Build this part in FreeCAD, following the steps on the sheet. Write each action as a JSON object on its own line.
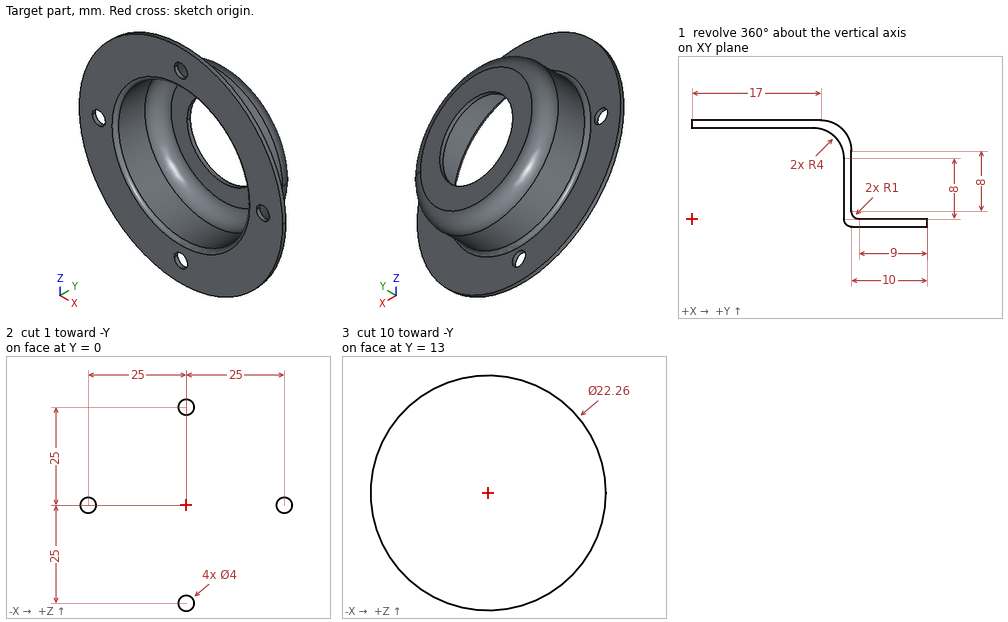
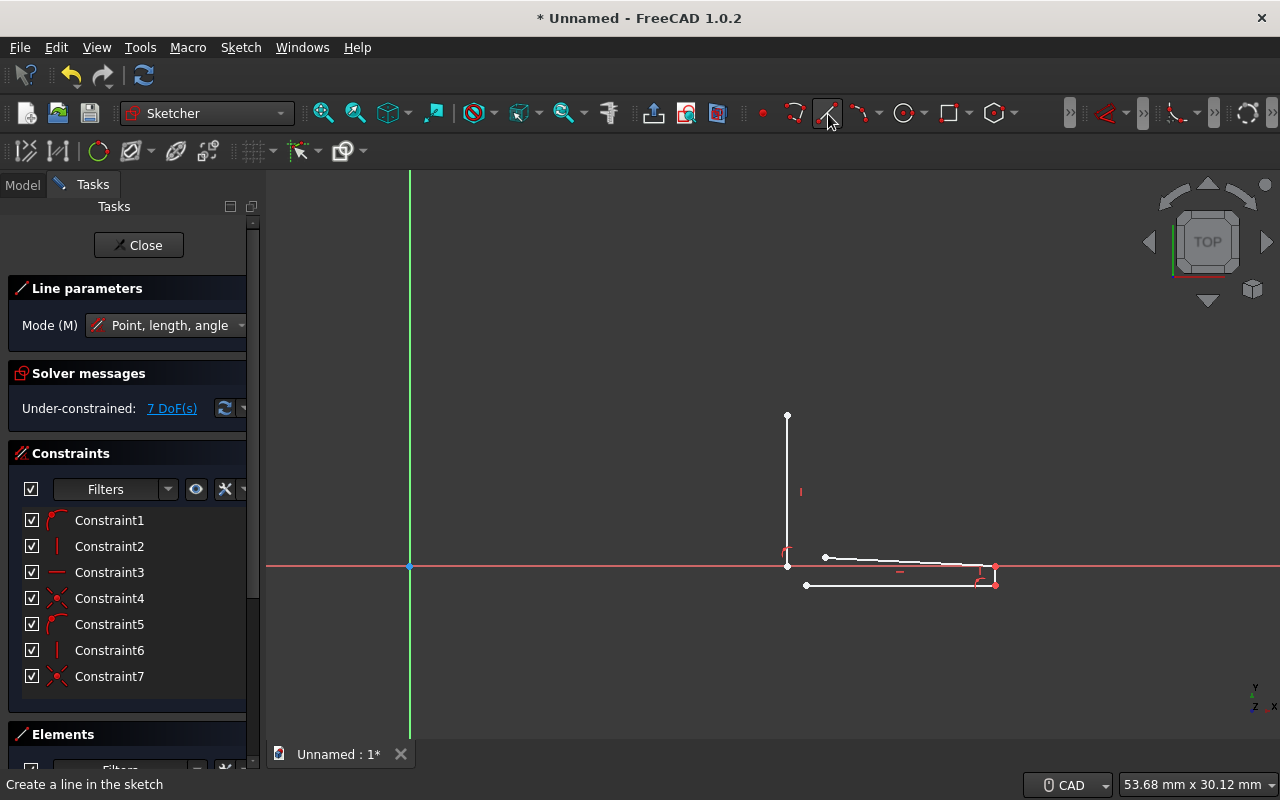
{"action": "left_click", "coordinate": [806, 547]}
{"action": "left_click", "coordinate": [806, 396]}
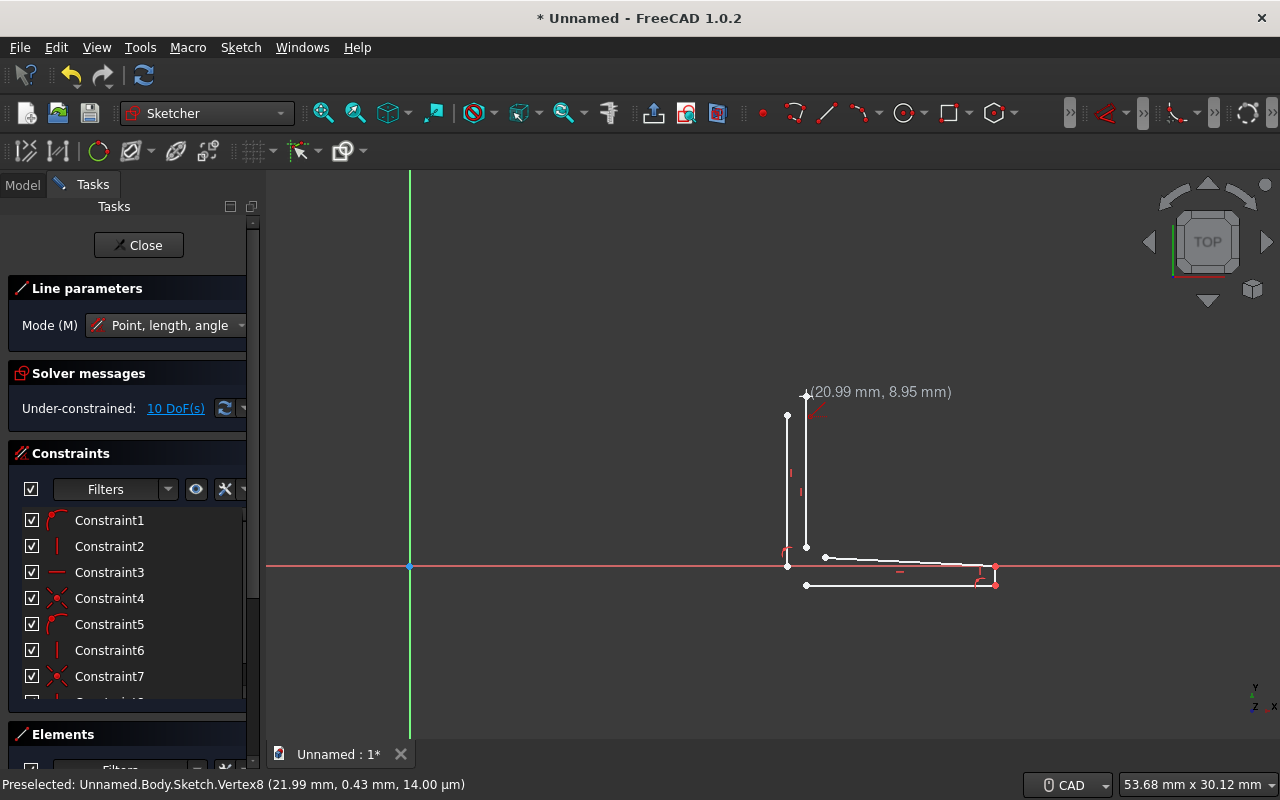
{"action": "left_click", "coordinate": [796, 114]}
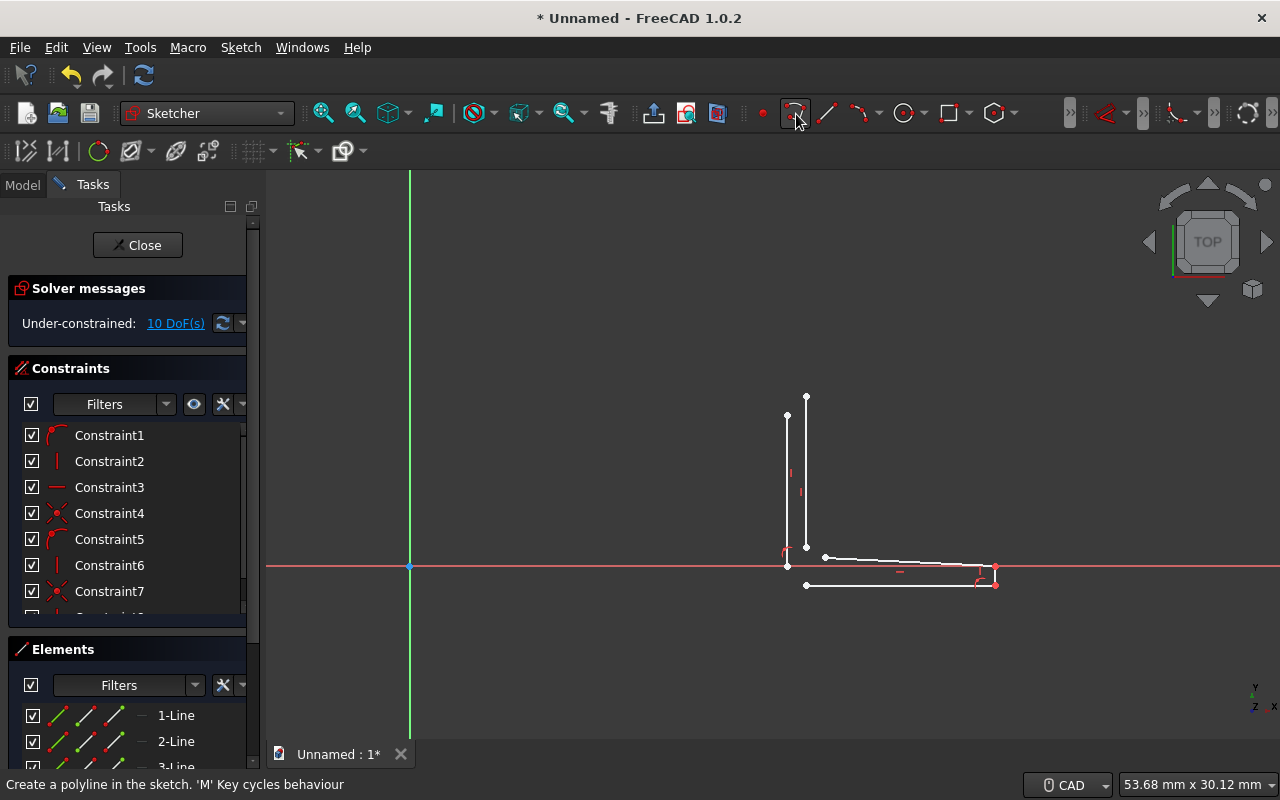
{"action": "left_click", "coordinate": [731, 320]}
{"action": "left_click", "coordinate": [410, 320]}
{"action": "left_click", "coordinate": [419, 339]}
{"action": "left_click", "coordinate": [712, 339]}
{"action": "right_click", "coordinate": [712, 339]}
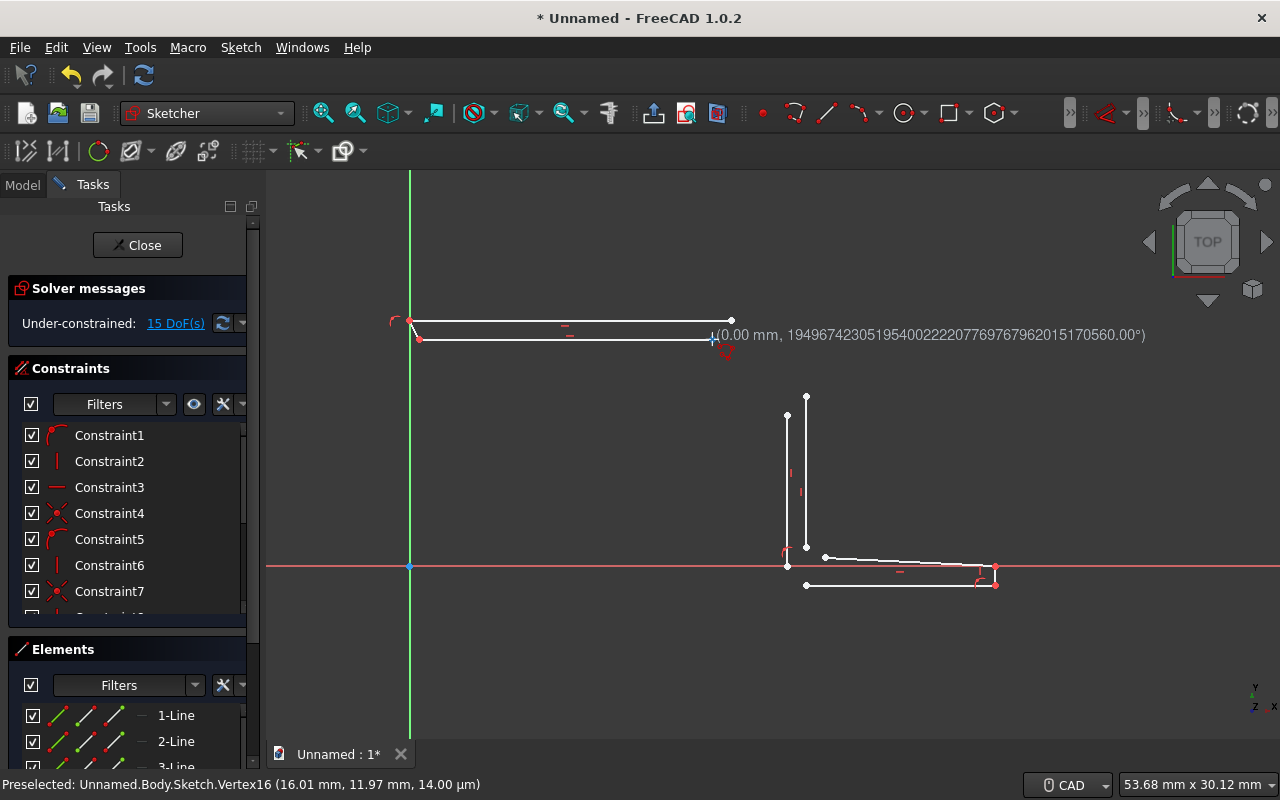
{"action": "left_click", "coordinate": [860, 114]}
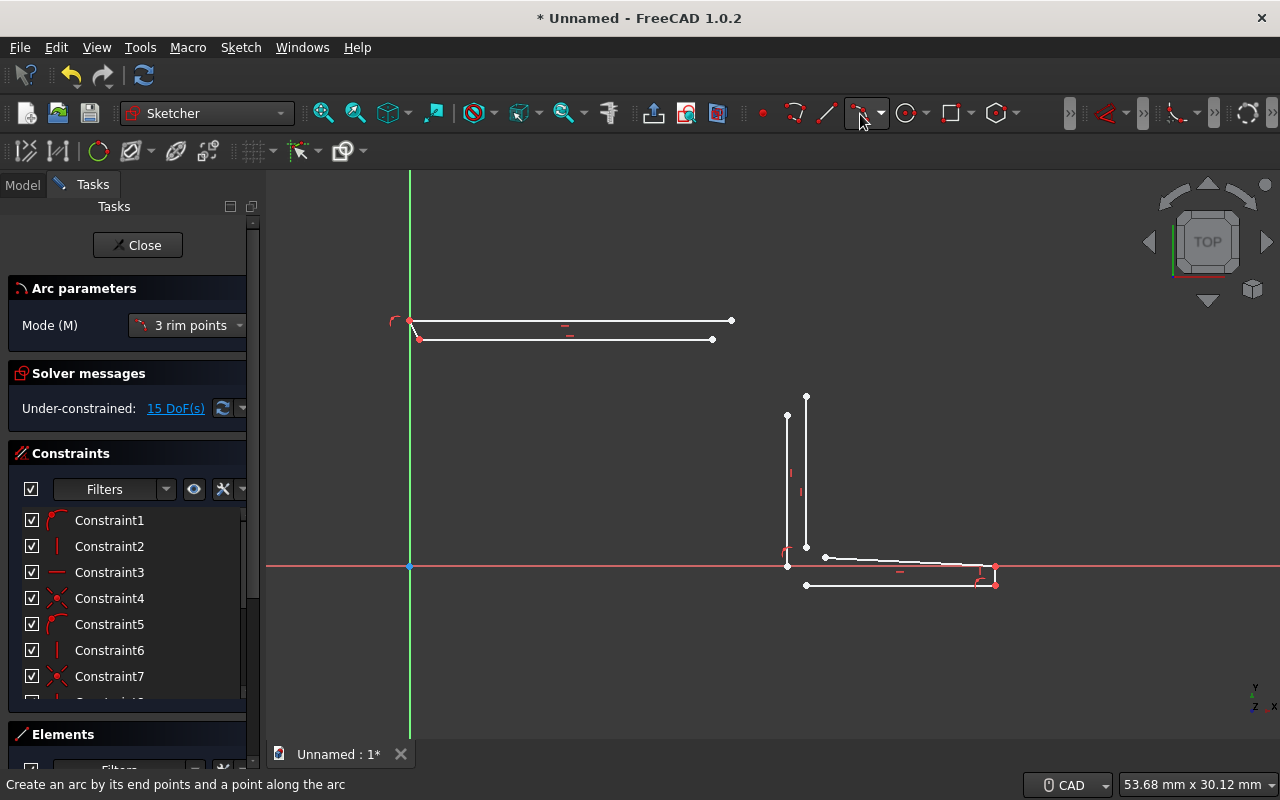
{"action": "left_click", "coordinate": [787, 566]}
{"action": "left_click", "coordinate": [806, 586]}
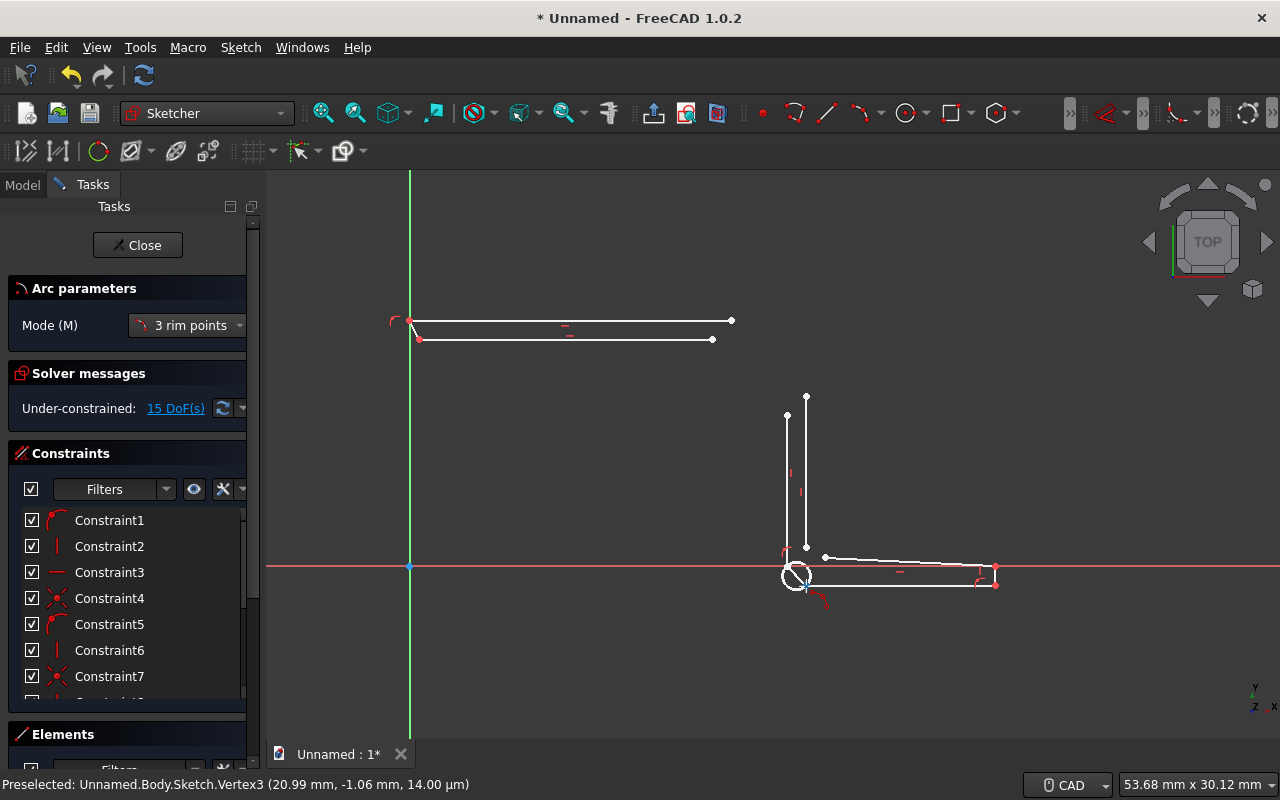
{"action": "scroll", "coordinate": [793, 579], "scroll_direction": "up", "scroll_amount": 6}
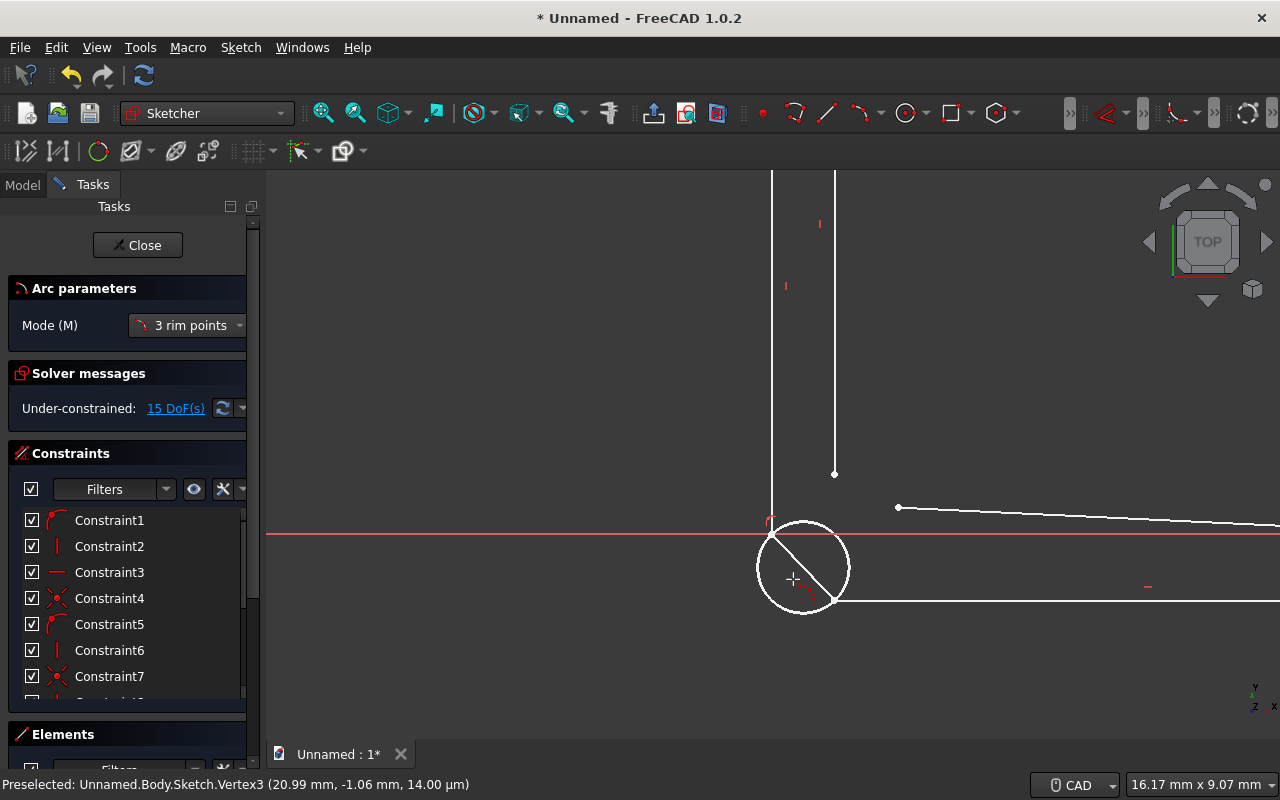
{"action": "left_click", "coordinate": [791, 579]}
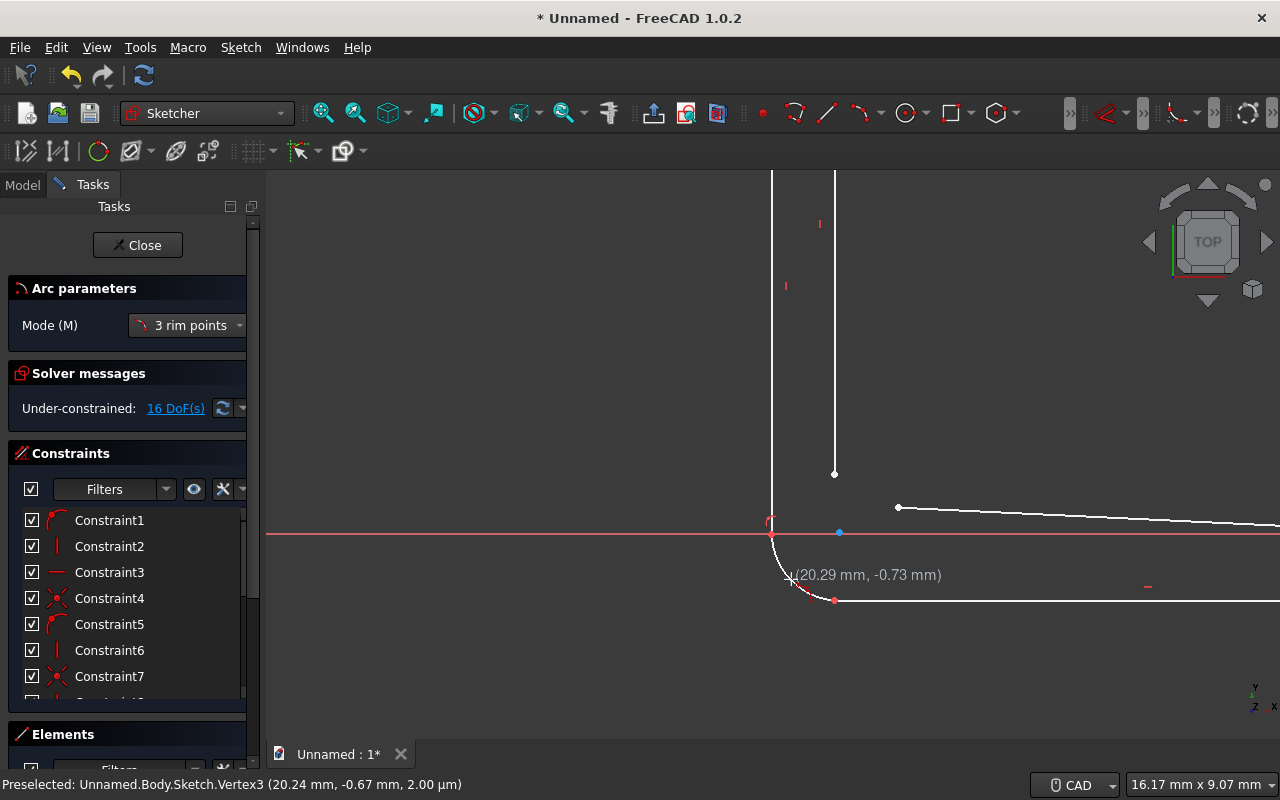
{"action": "left_click", "coordinate": [898, 508]}
{"action": "left_click", "coordinate": [835, 474]}
{"action": "left_click", "coordinate": [854, 516]}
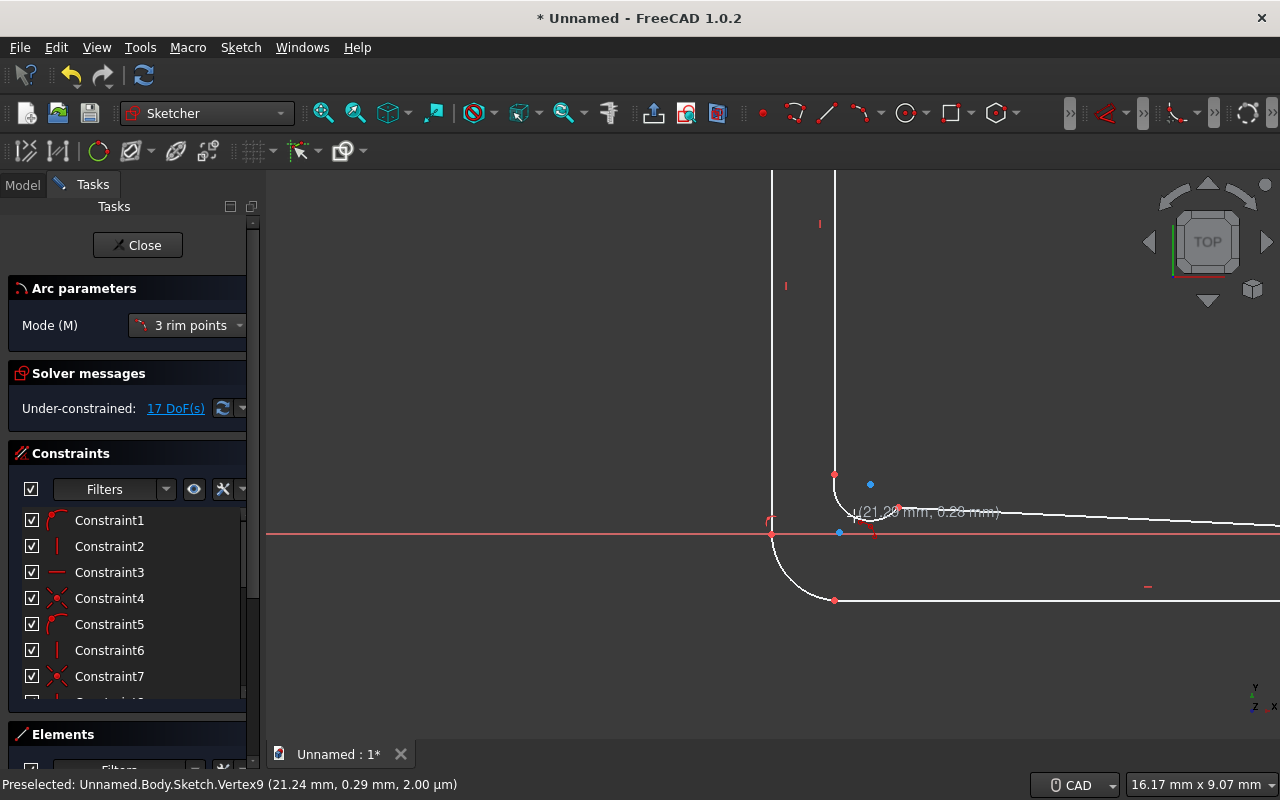
{"action": "scroll", "coordinate": [797, 582], "scroll_direction": "down", "scroll_amount": 6}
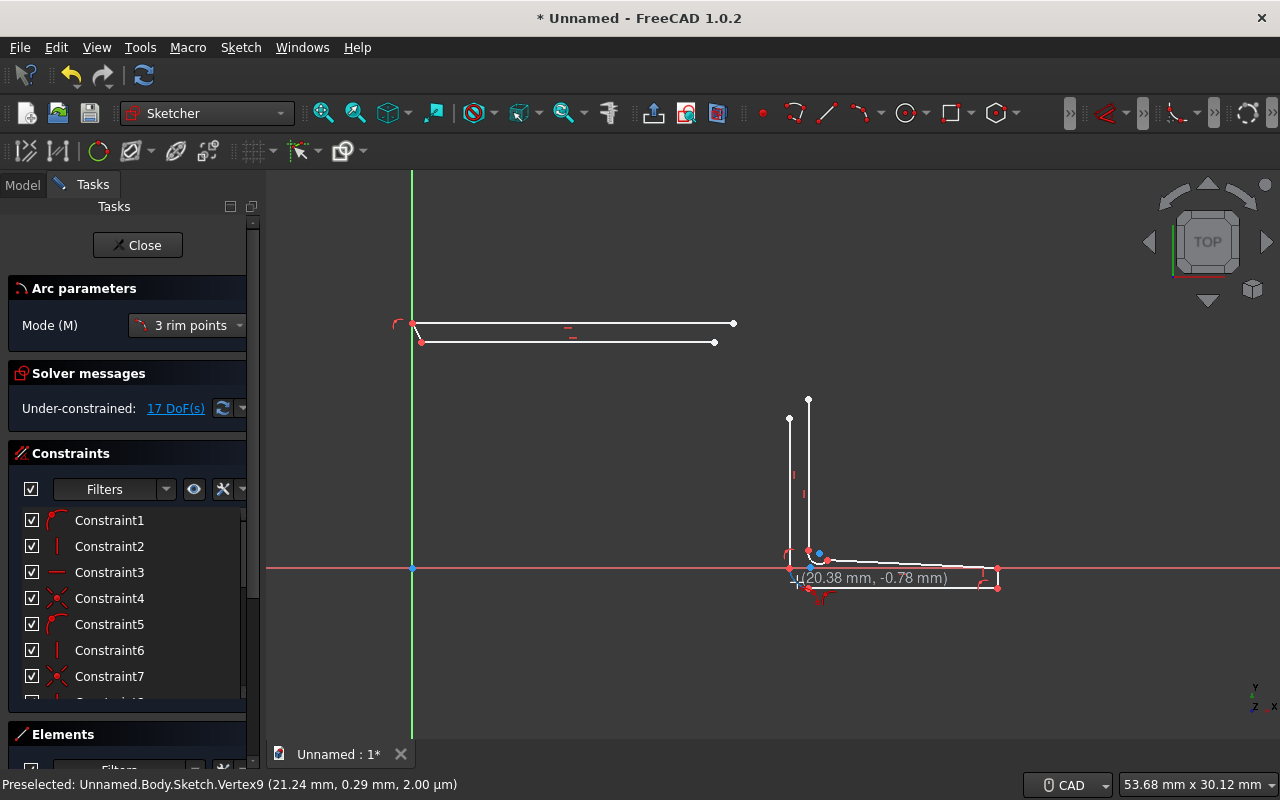
{"action": "left_click", "coordinate": [809, 399]}
{"action": "left_click", "coordinate": [734, 323]}
{"action": "left_click", "coordinate": [787, 345]}